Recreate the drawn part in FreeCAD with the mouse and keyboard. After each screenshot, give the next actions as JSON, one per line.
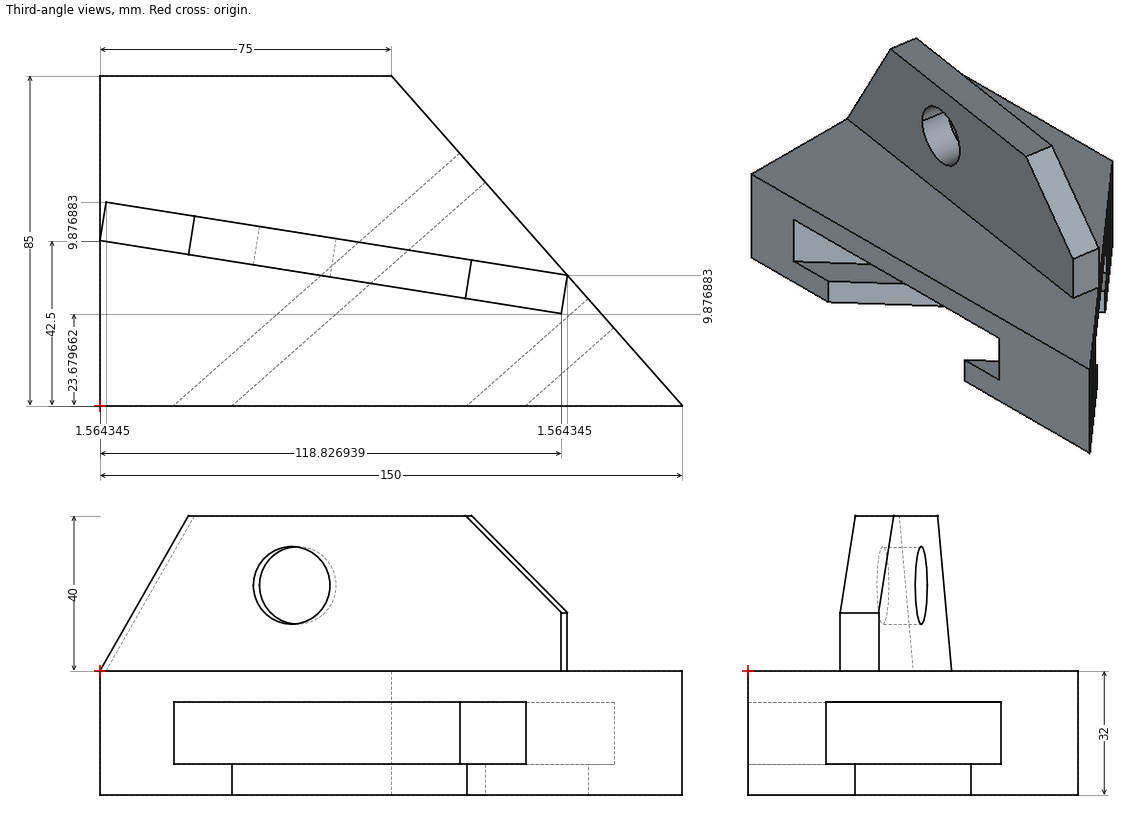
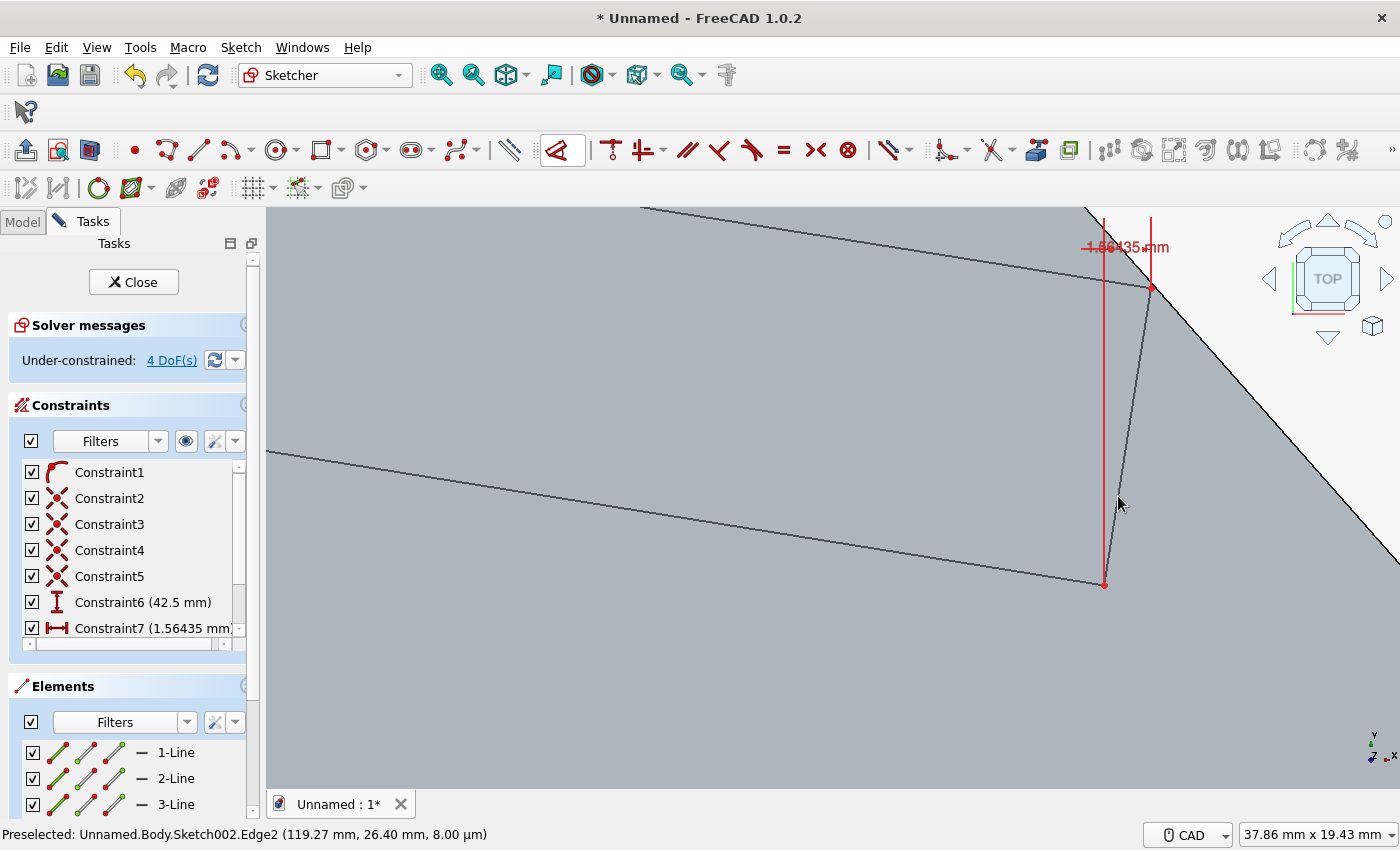
{"action": "scroll", "coordinate": [1123, 497], "scroll_direction": "down", "scroll_amount": 8}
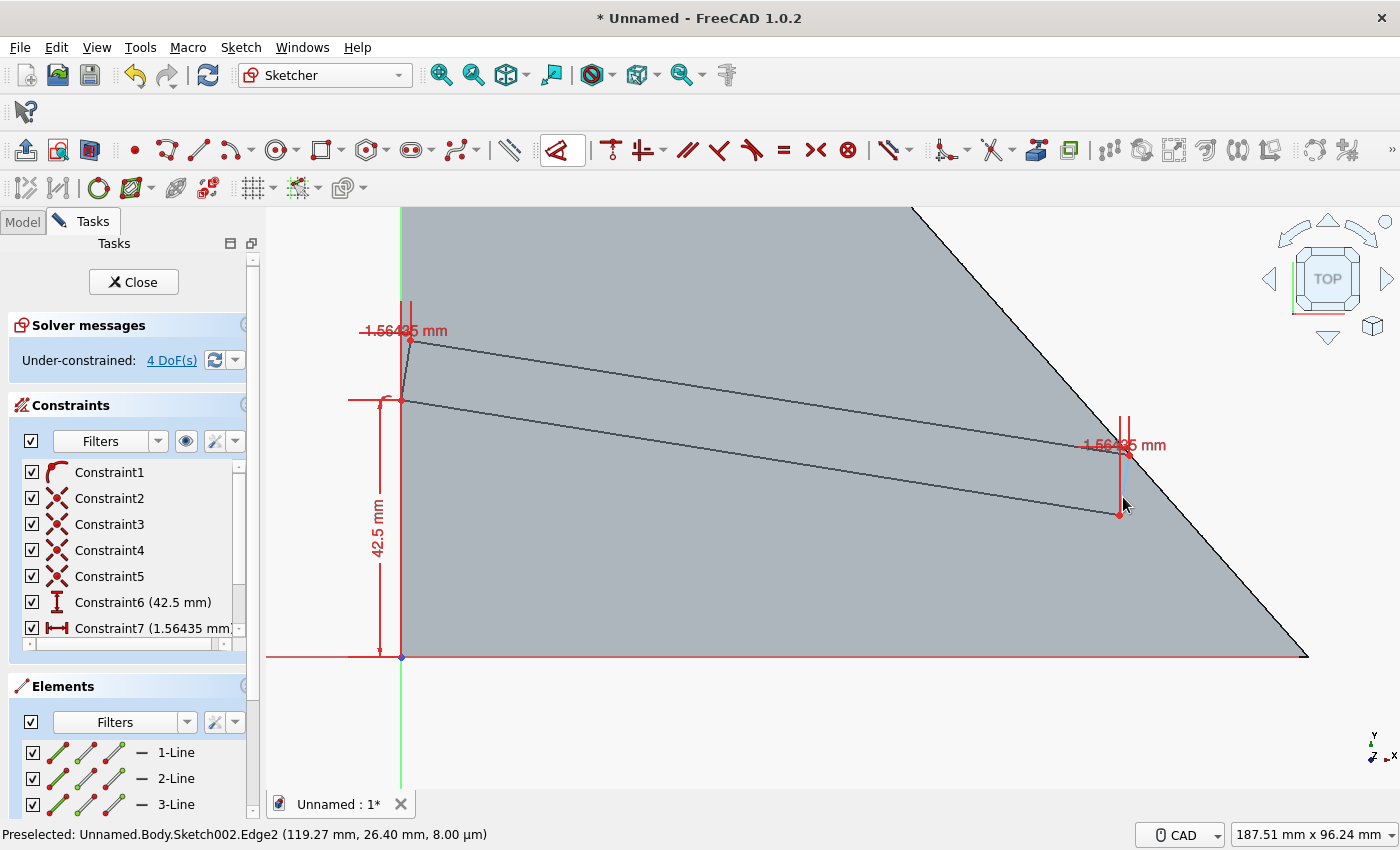
{"action": "left_click", "coordinate": [1123, 497]}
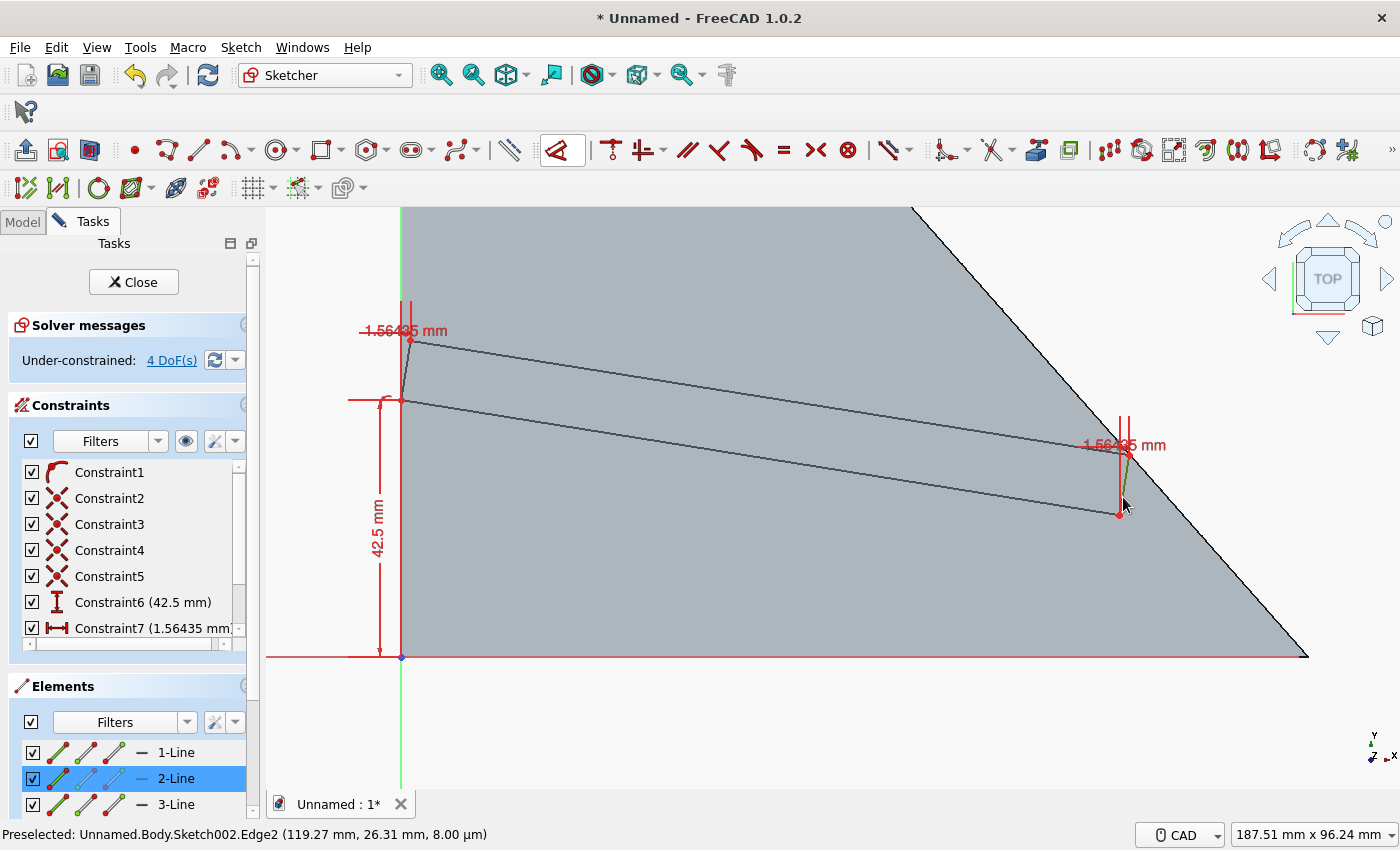
{"action": "key", "text": "i"}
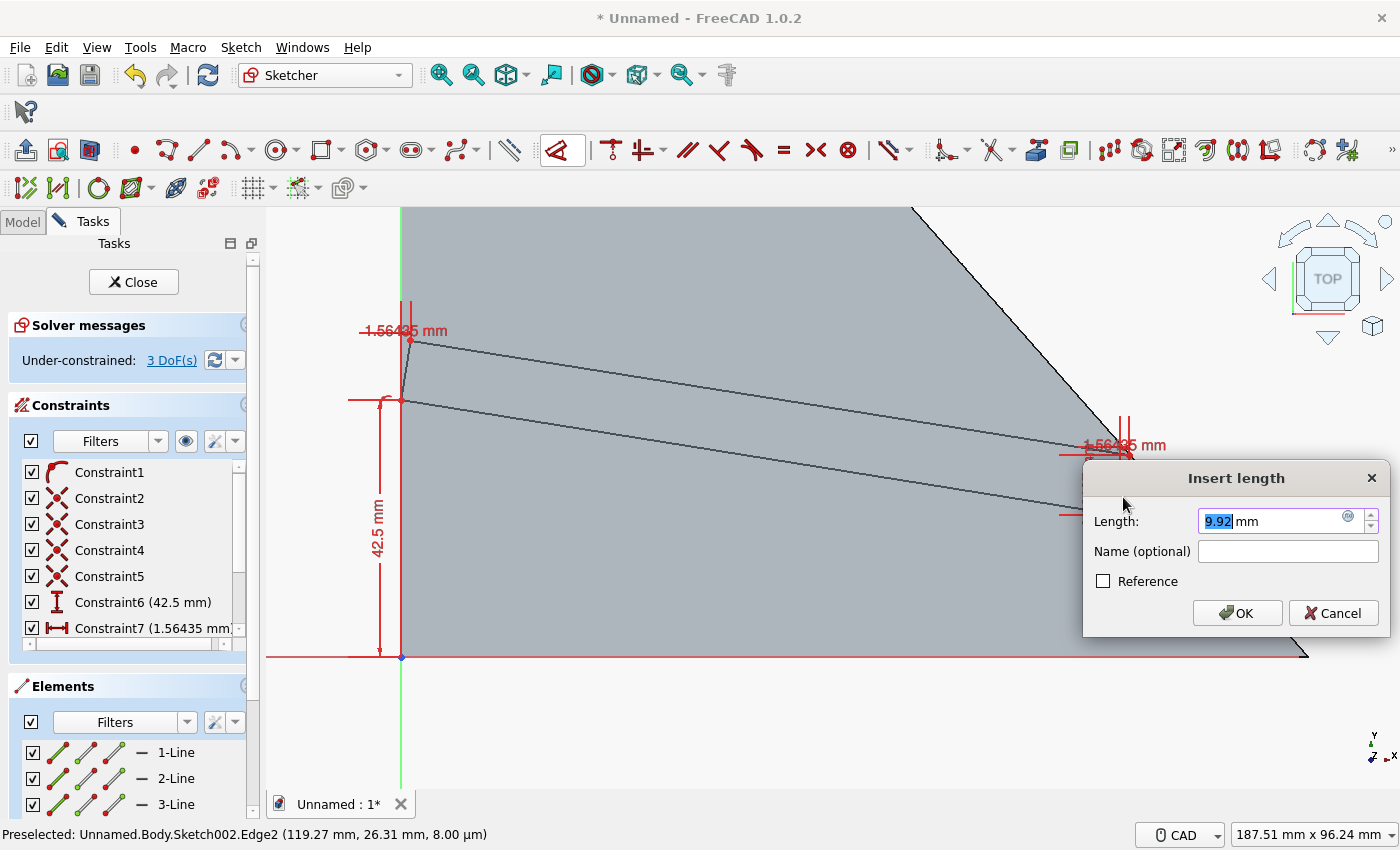
{"action": "type", "text": "9.876883"}
{"action": "key", "text": "Return"}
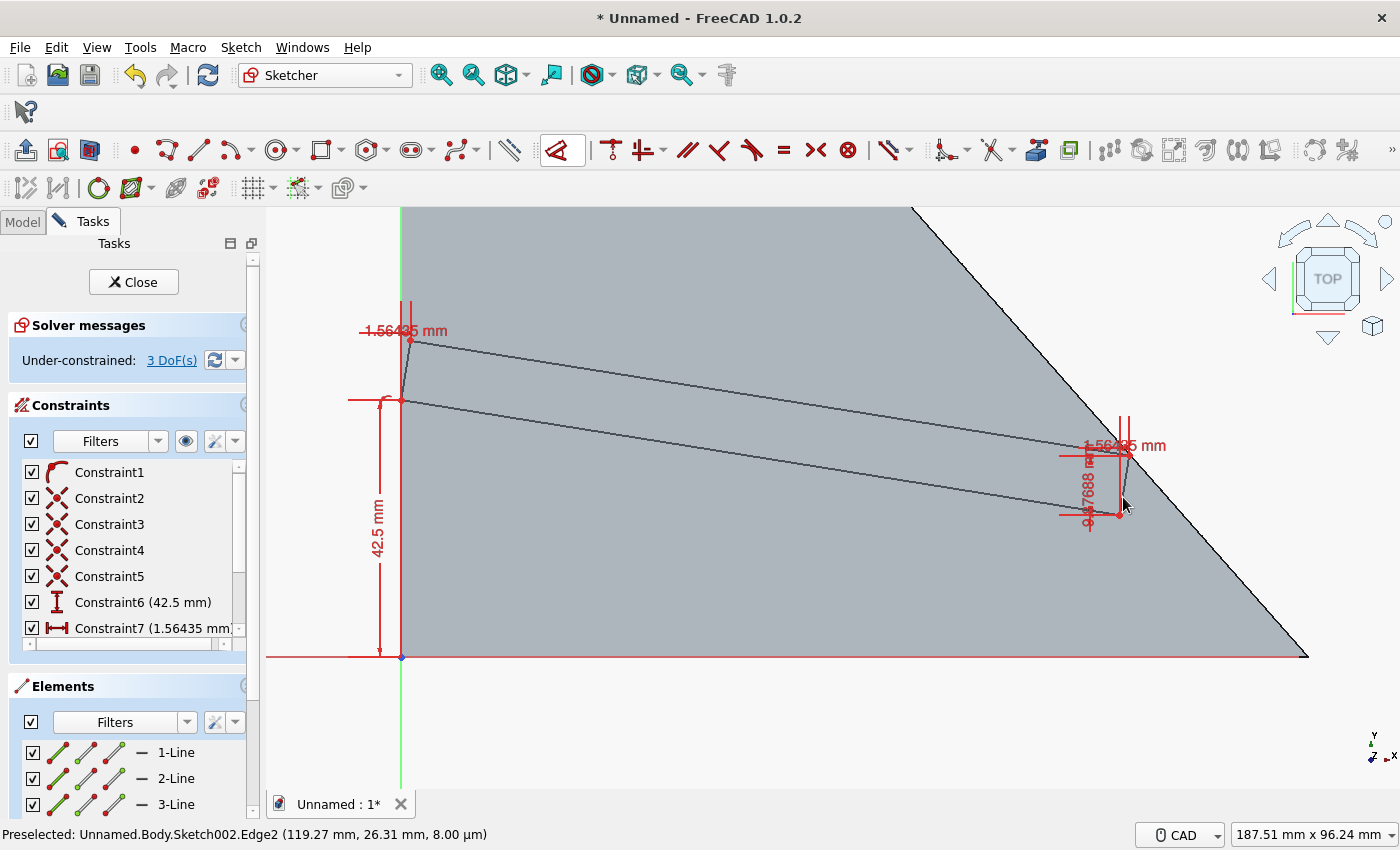
{"action": "left_click", "coordinate": [404, 382]}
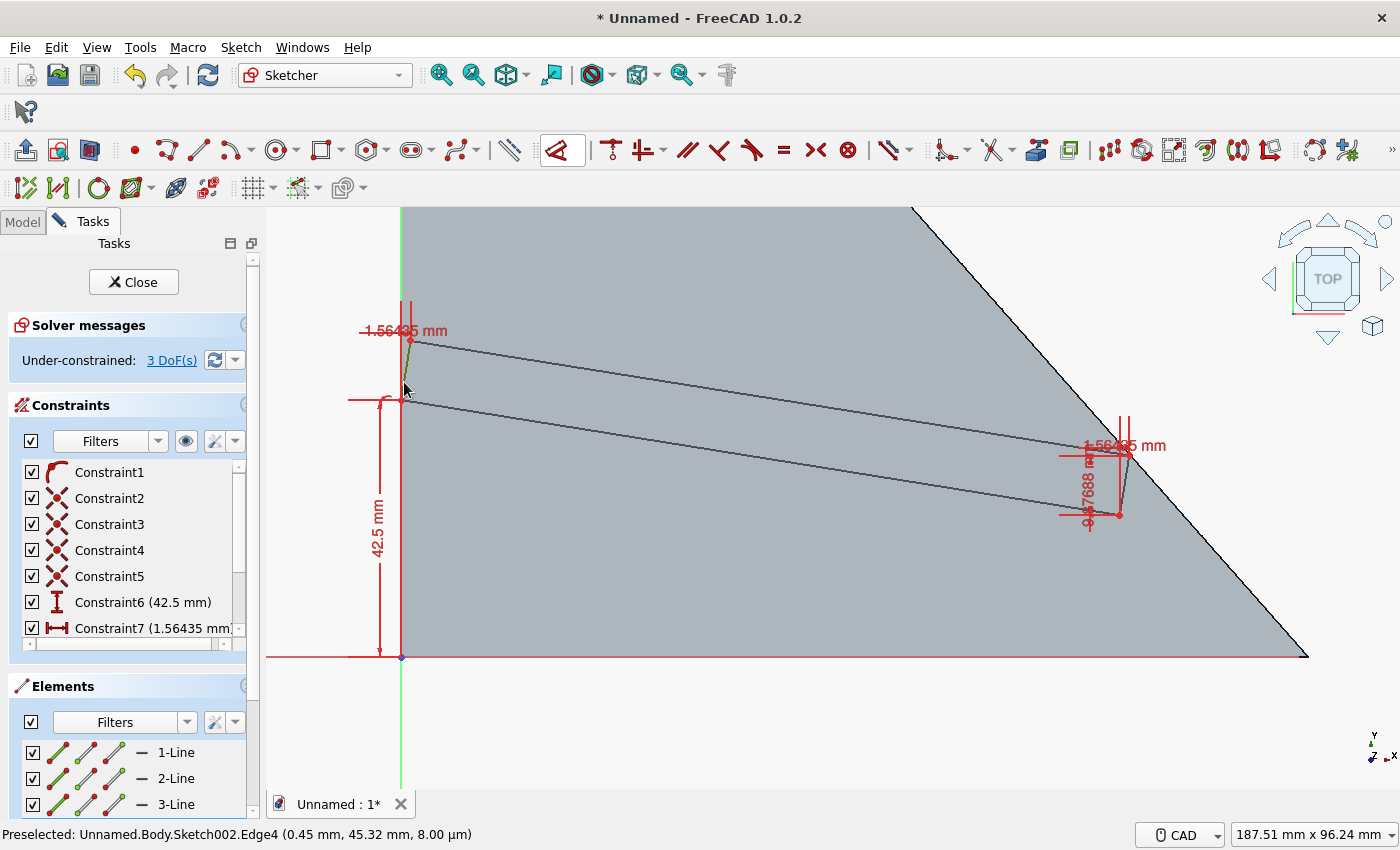
{"action": "key", "text": "i"}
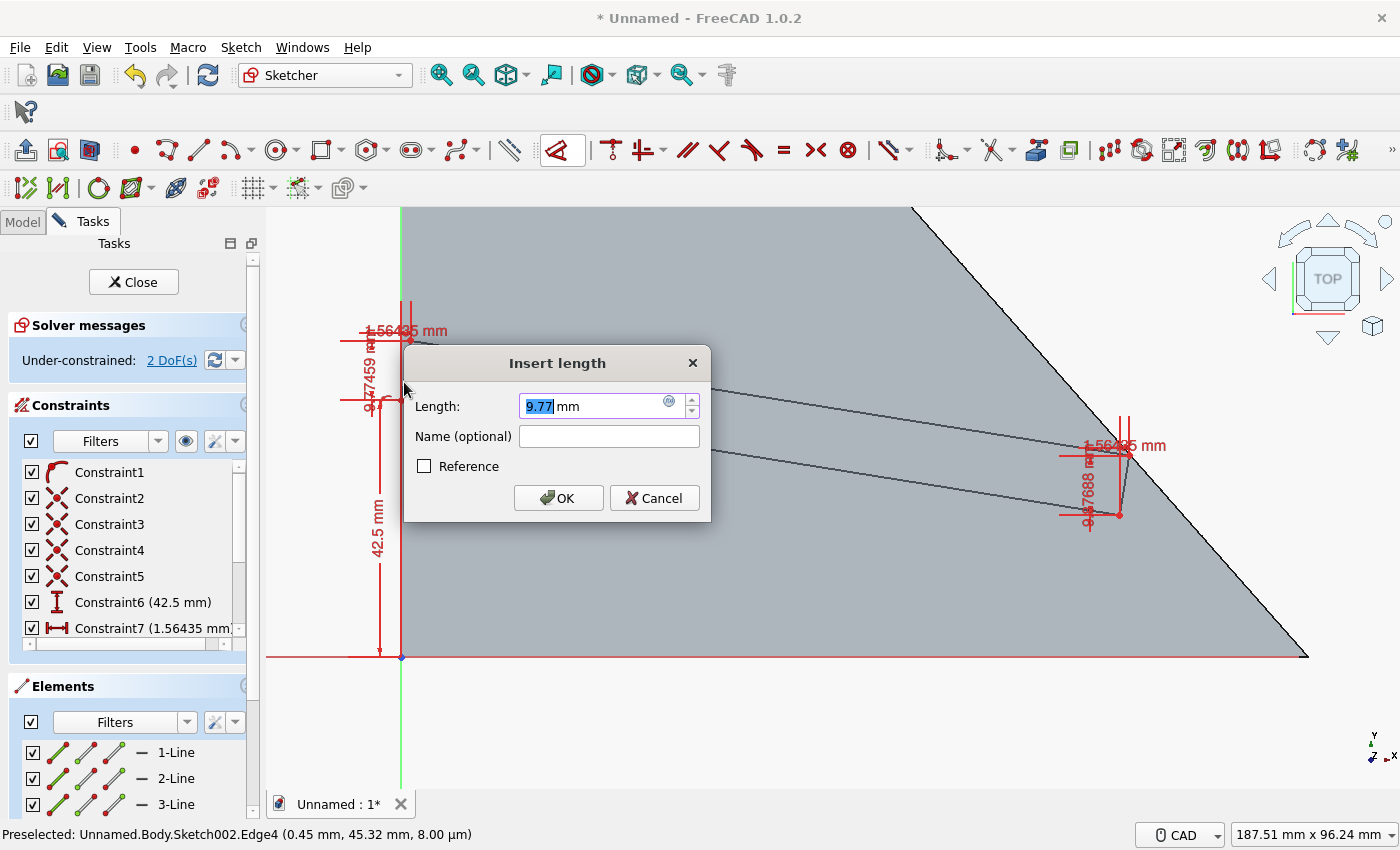
{"action": "type", "text": "9.876883"}
{"action": "key", "text": "Return"}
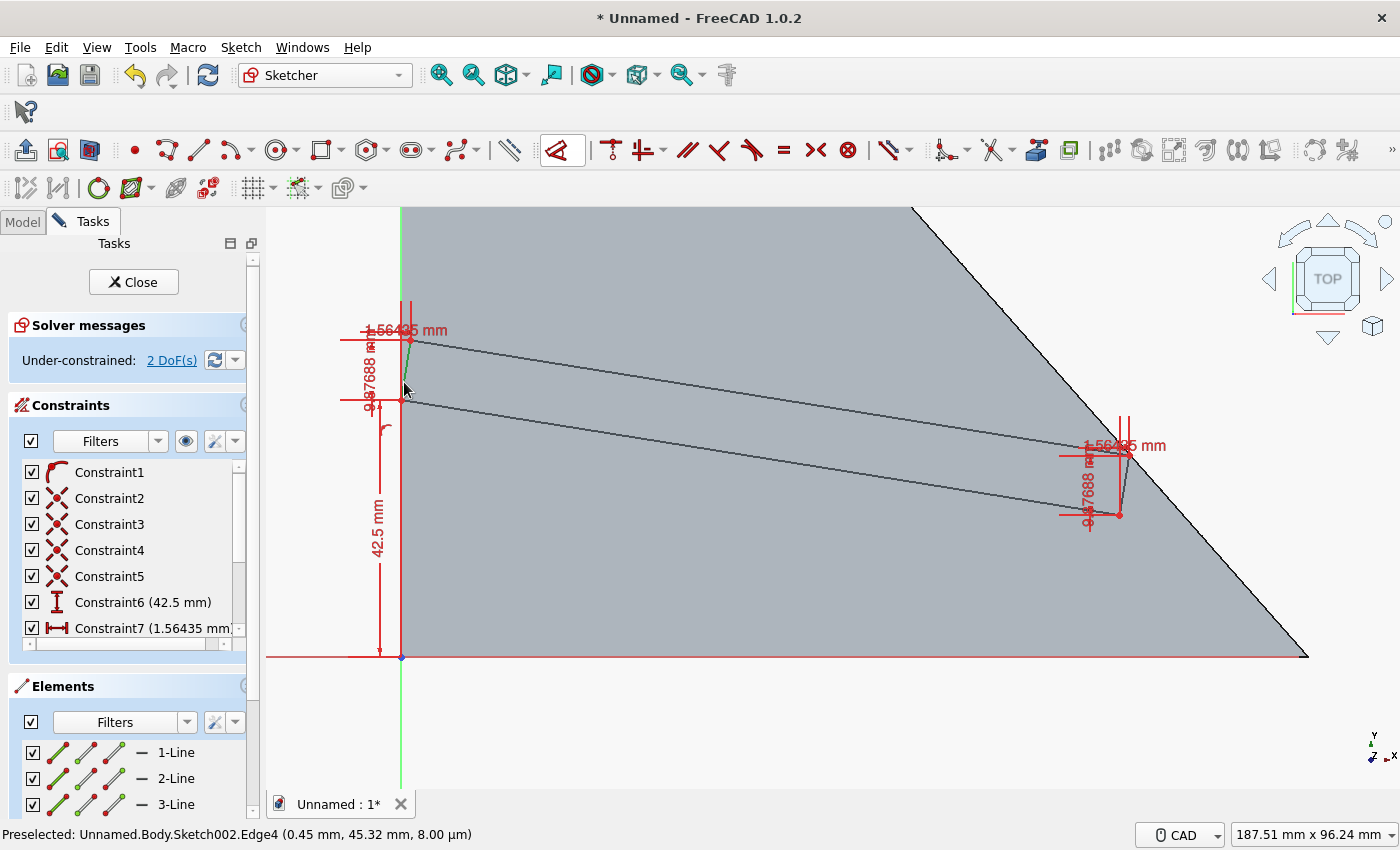
{"action": "left_click", "coordinate": [1120, 515]}